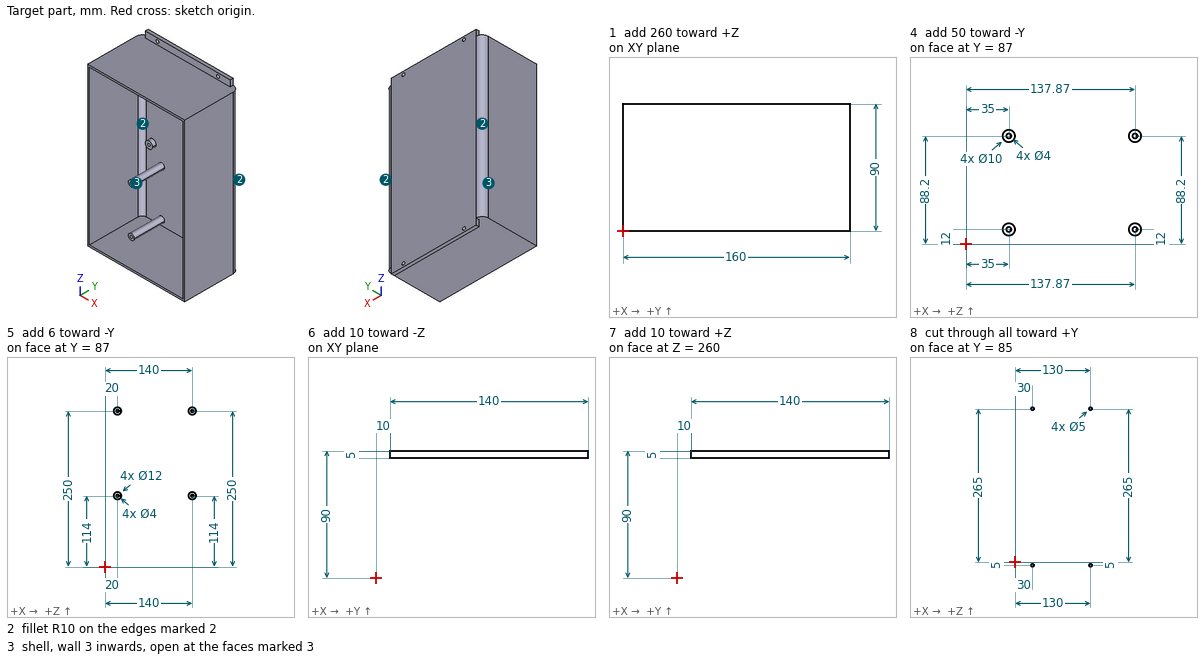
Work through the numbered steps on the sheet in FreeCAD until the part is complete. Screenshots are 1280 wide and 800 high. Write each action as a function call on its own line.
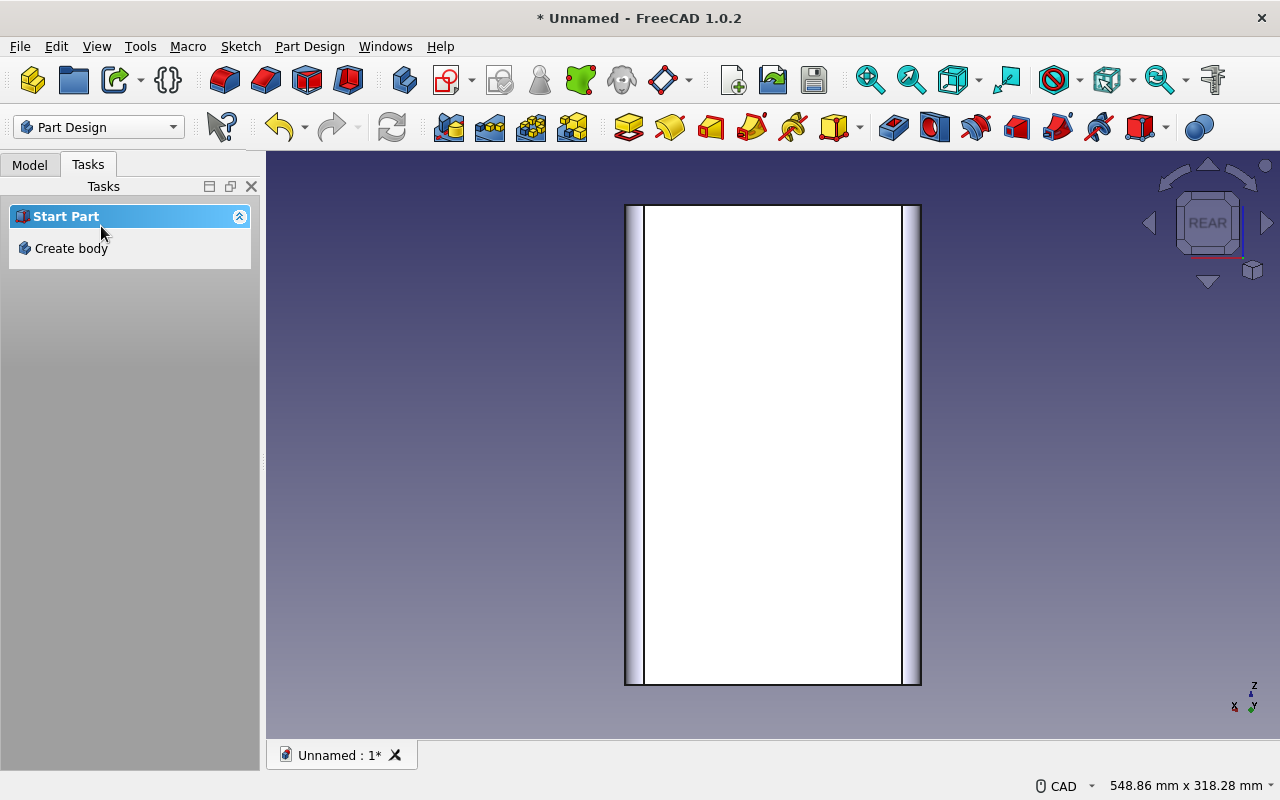
key(0)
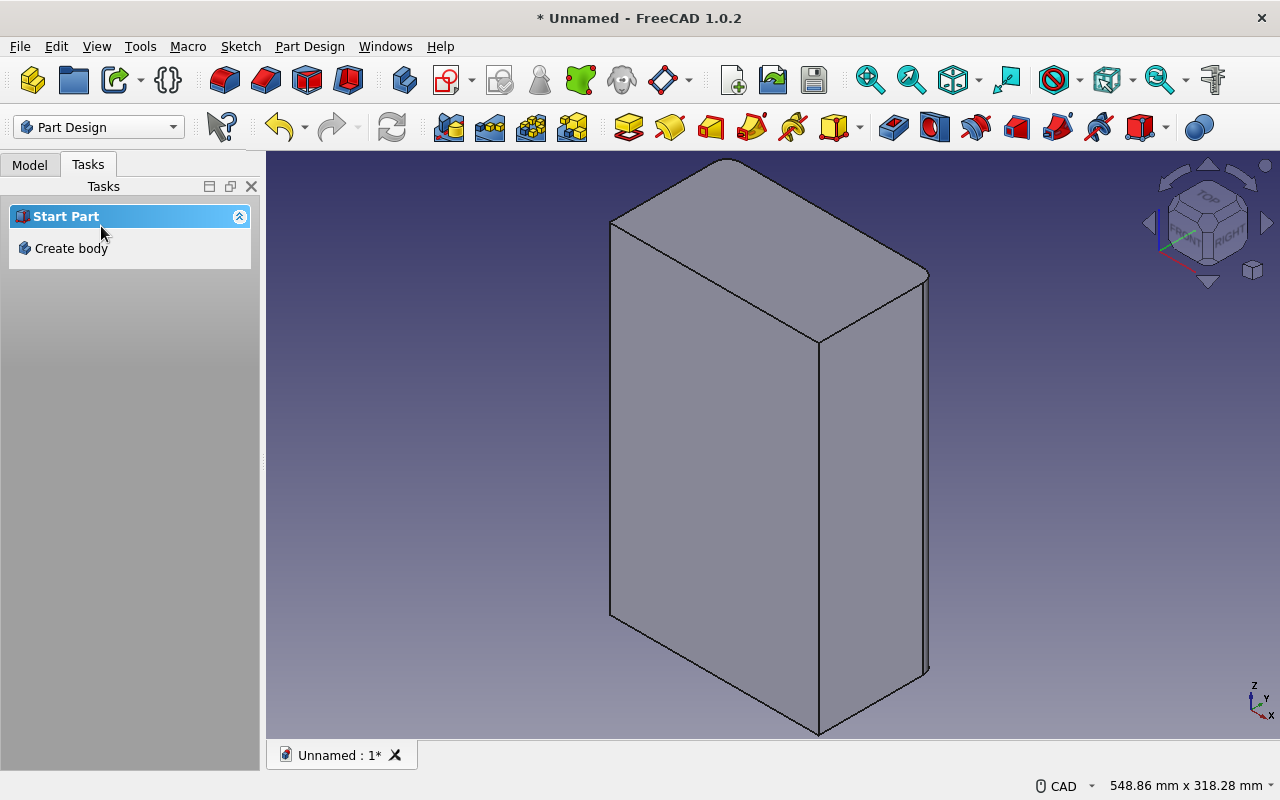
click(714, 422)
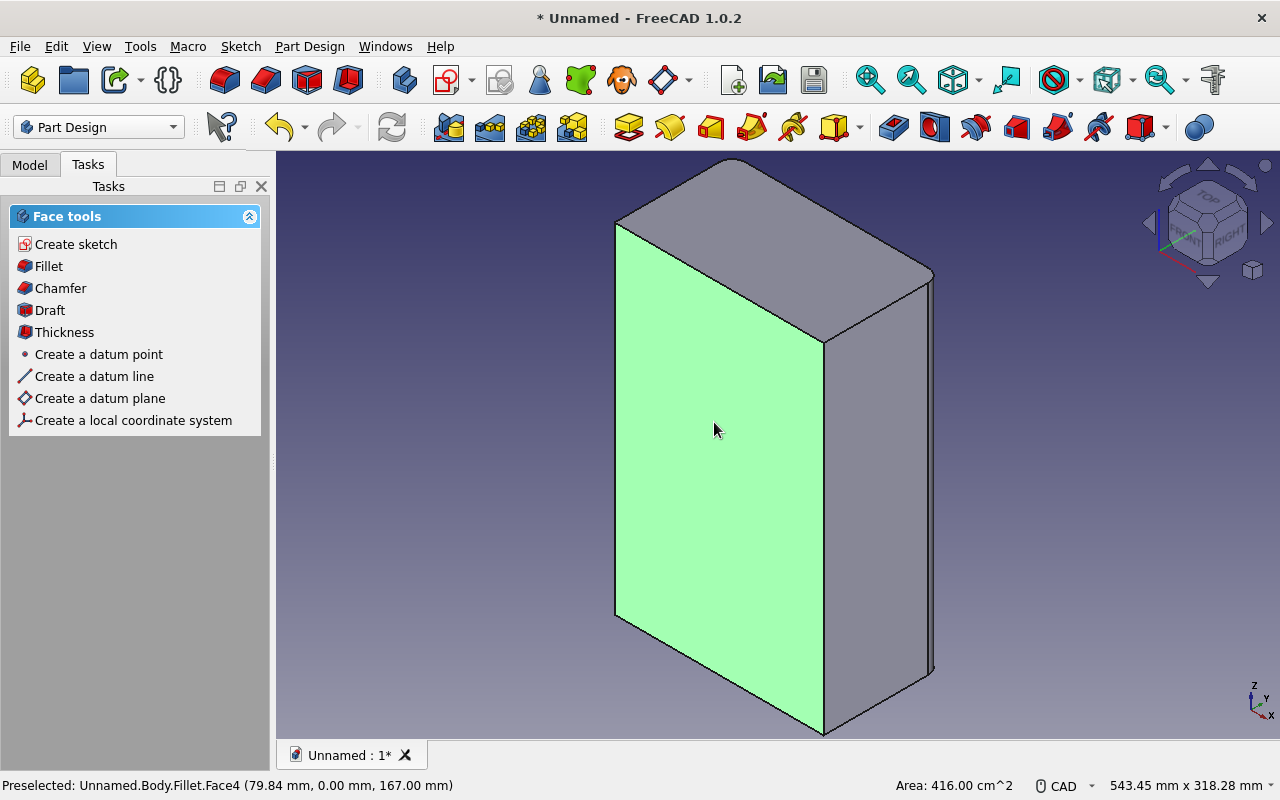
click(348, 80)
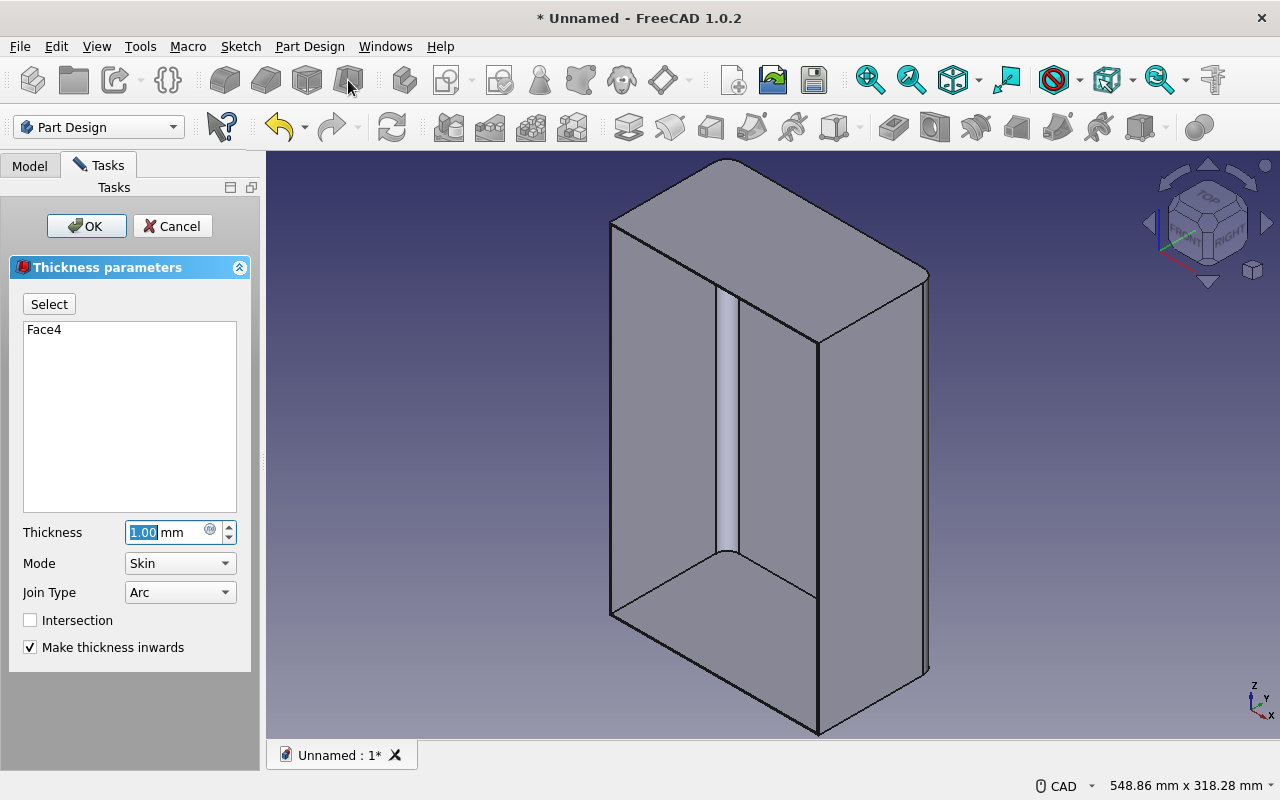
text(3)
key(Tab)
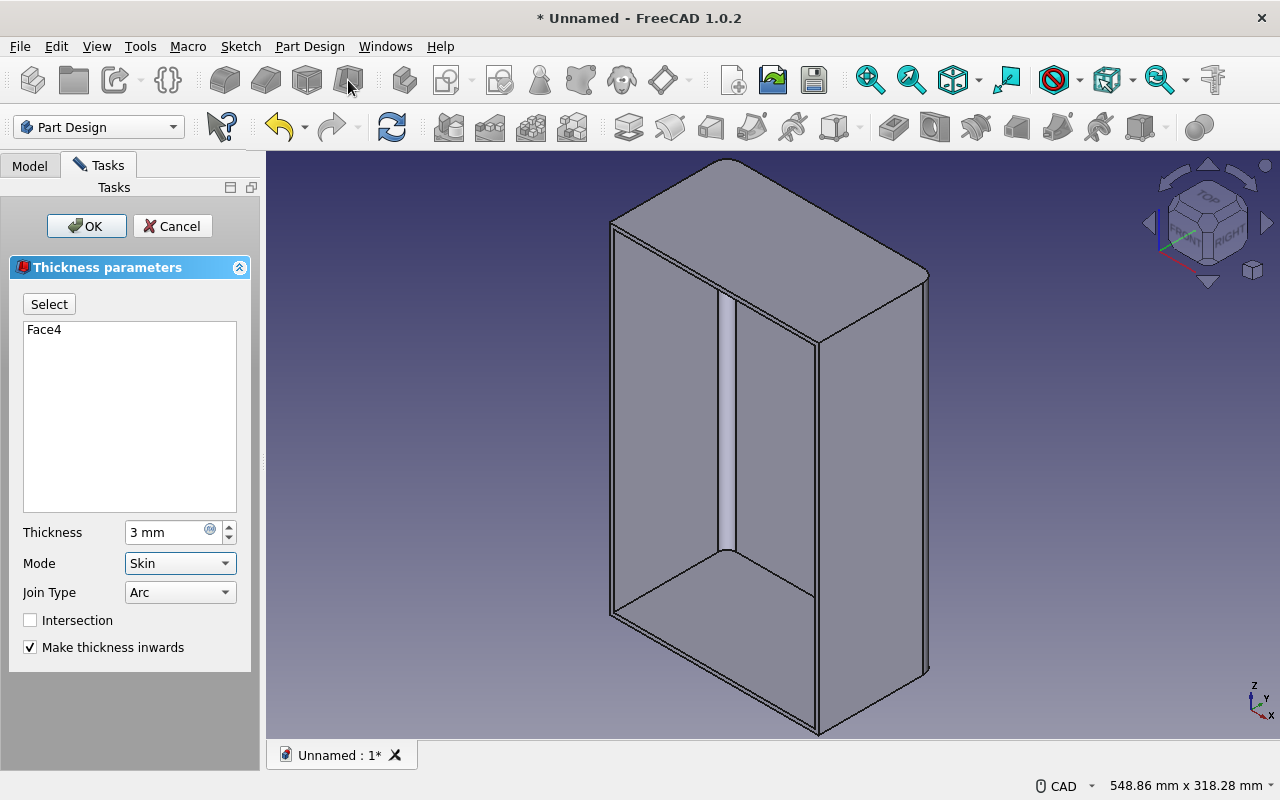
click(181, 592)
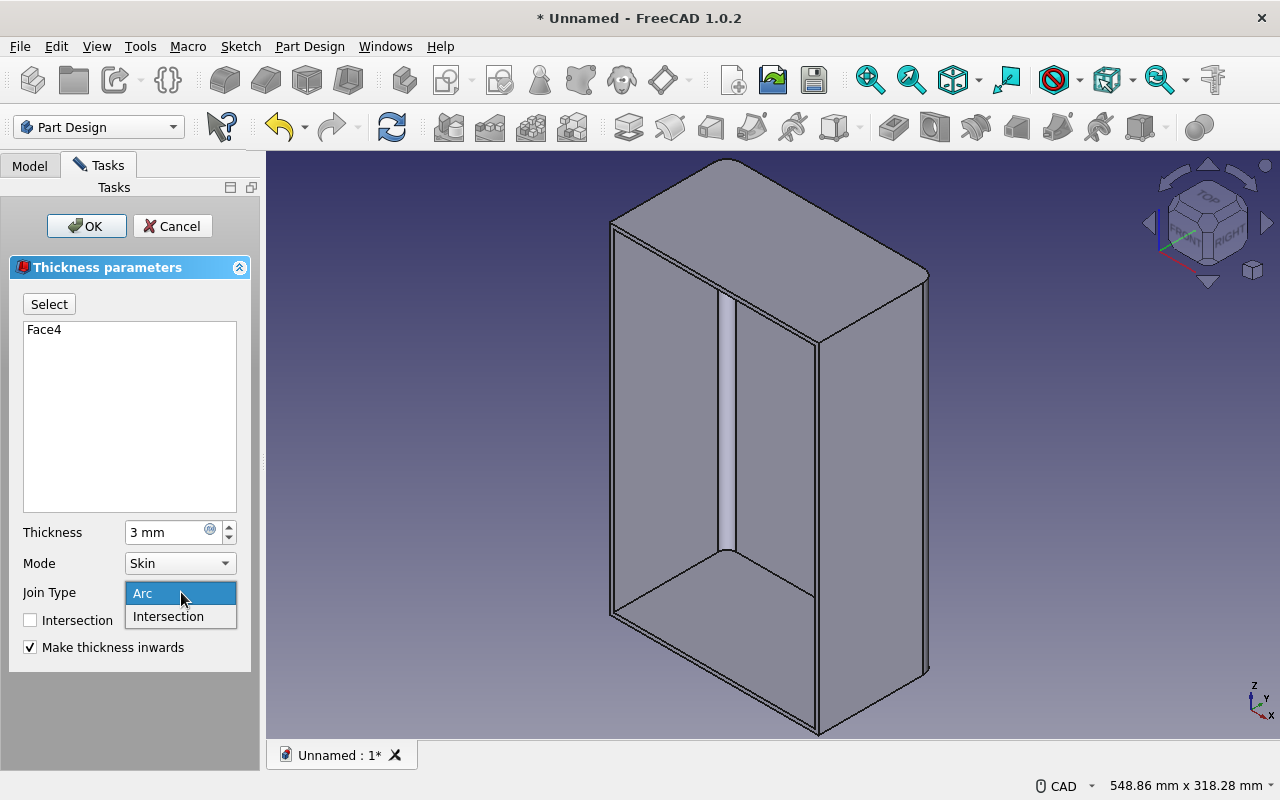
click(179, 616)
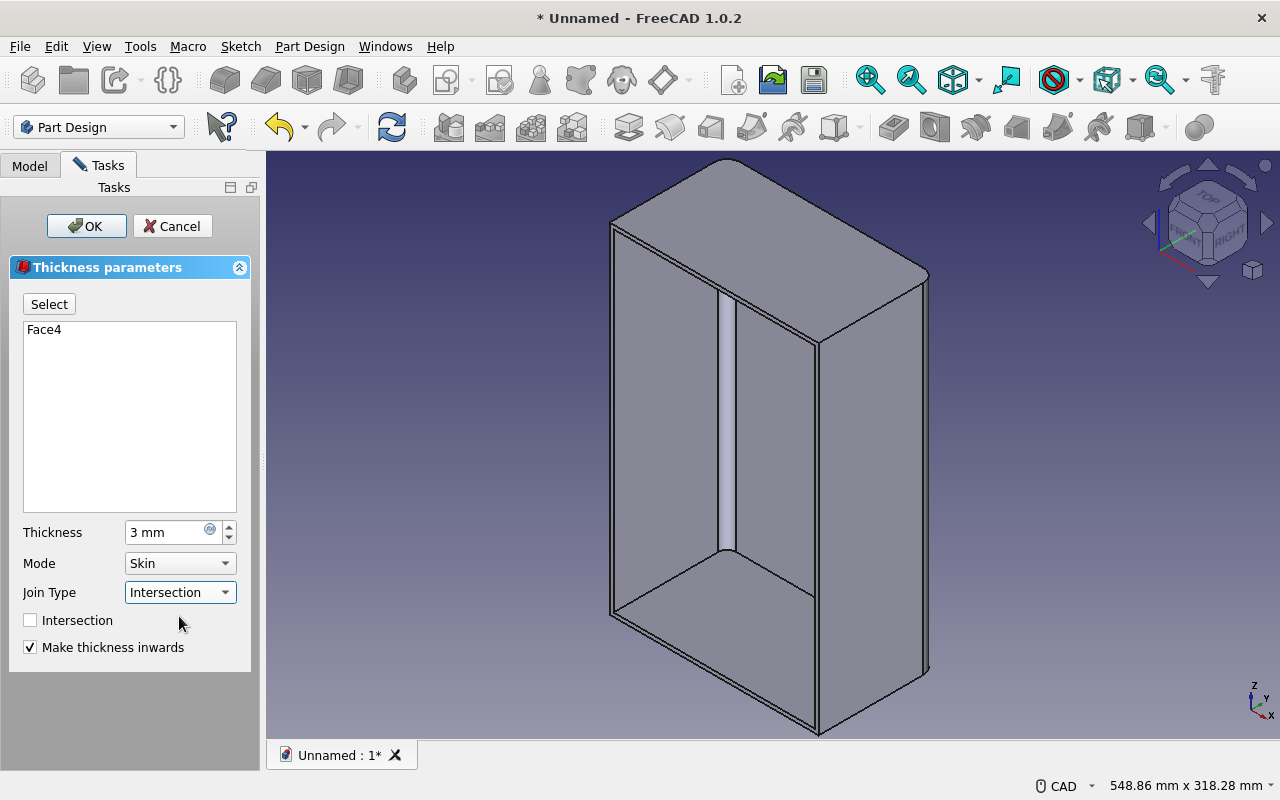
click(87, 226)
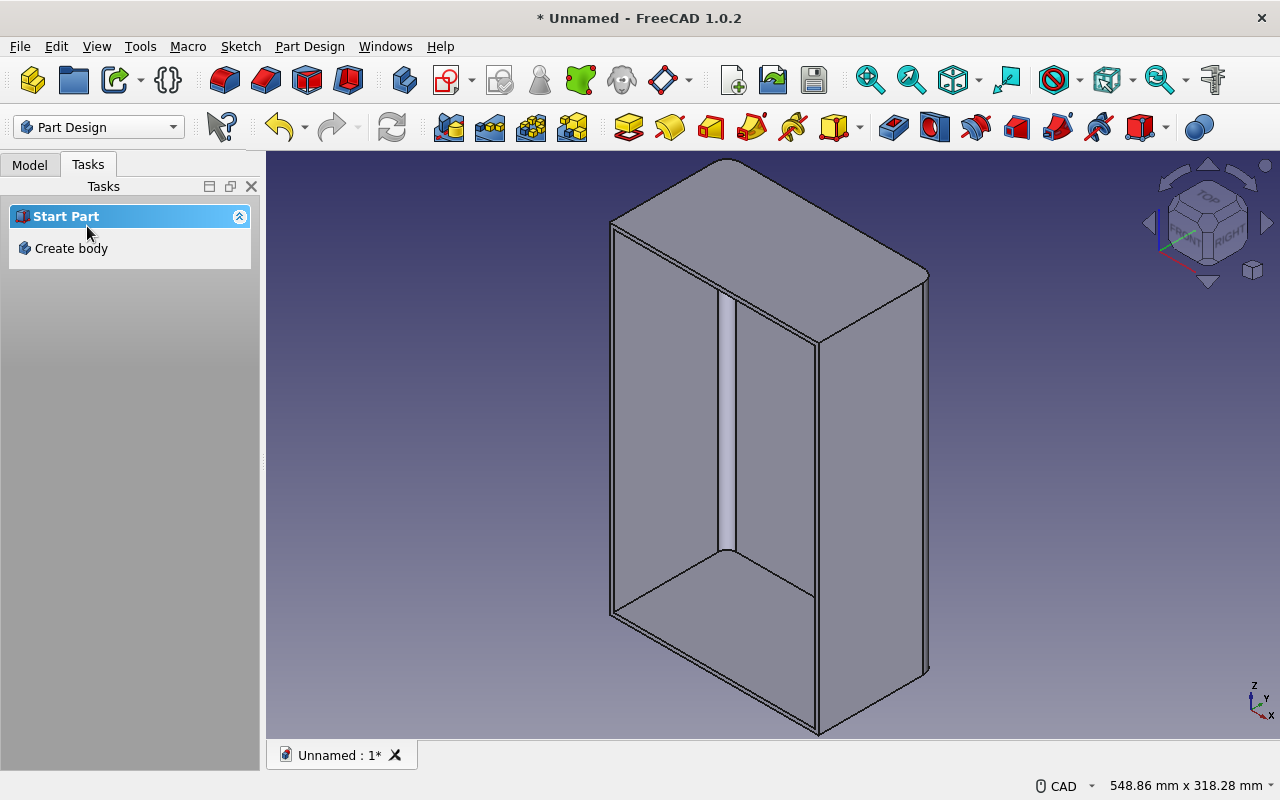
key(1)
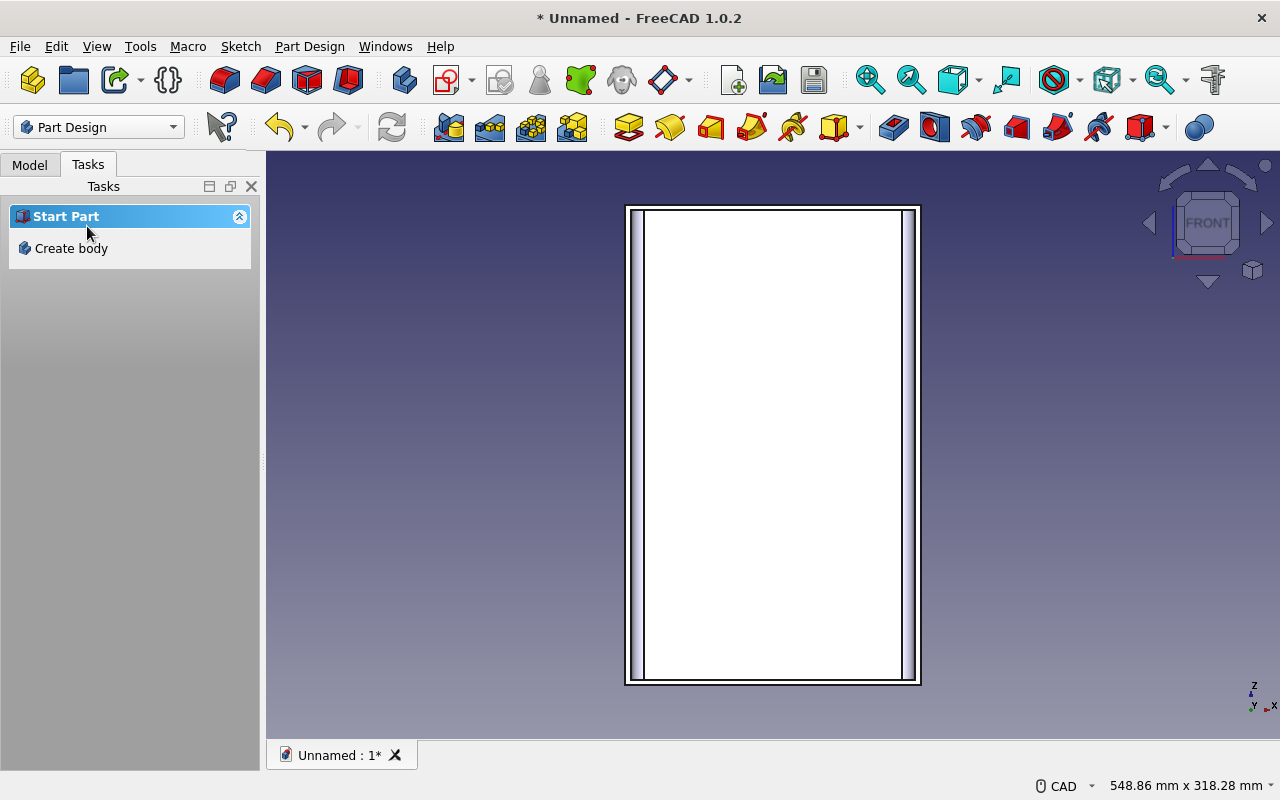
click(773, 377)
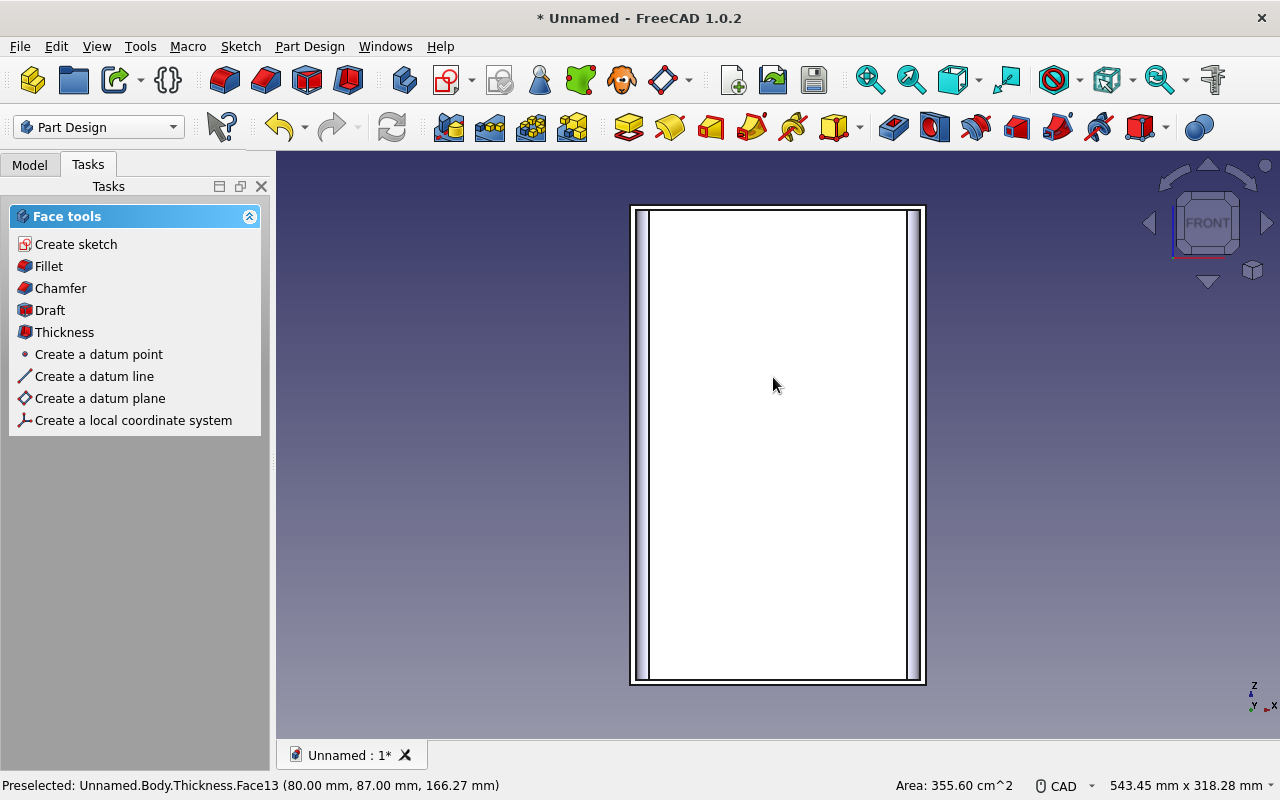
click(446, 80)